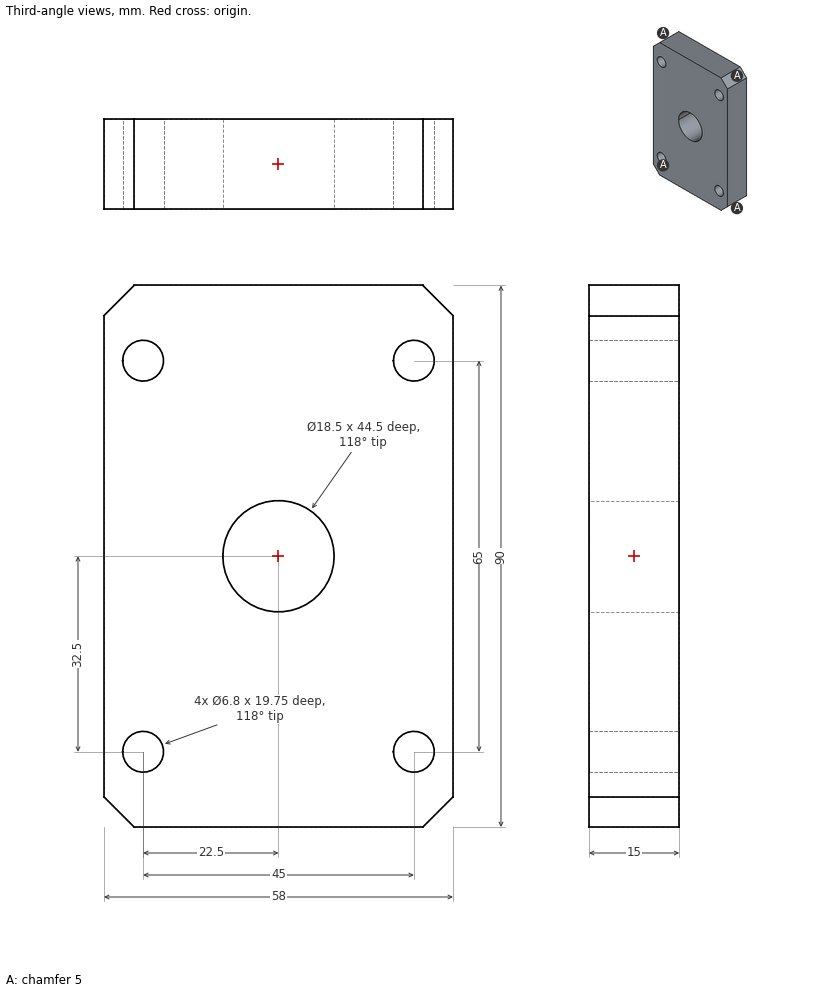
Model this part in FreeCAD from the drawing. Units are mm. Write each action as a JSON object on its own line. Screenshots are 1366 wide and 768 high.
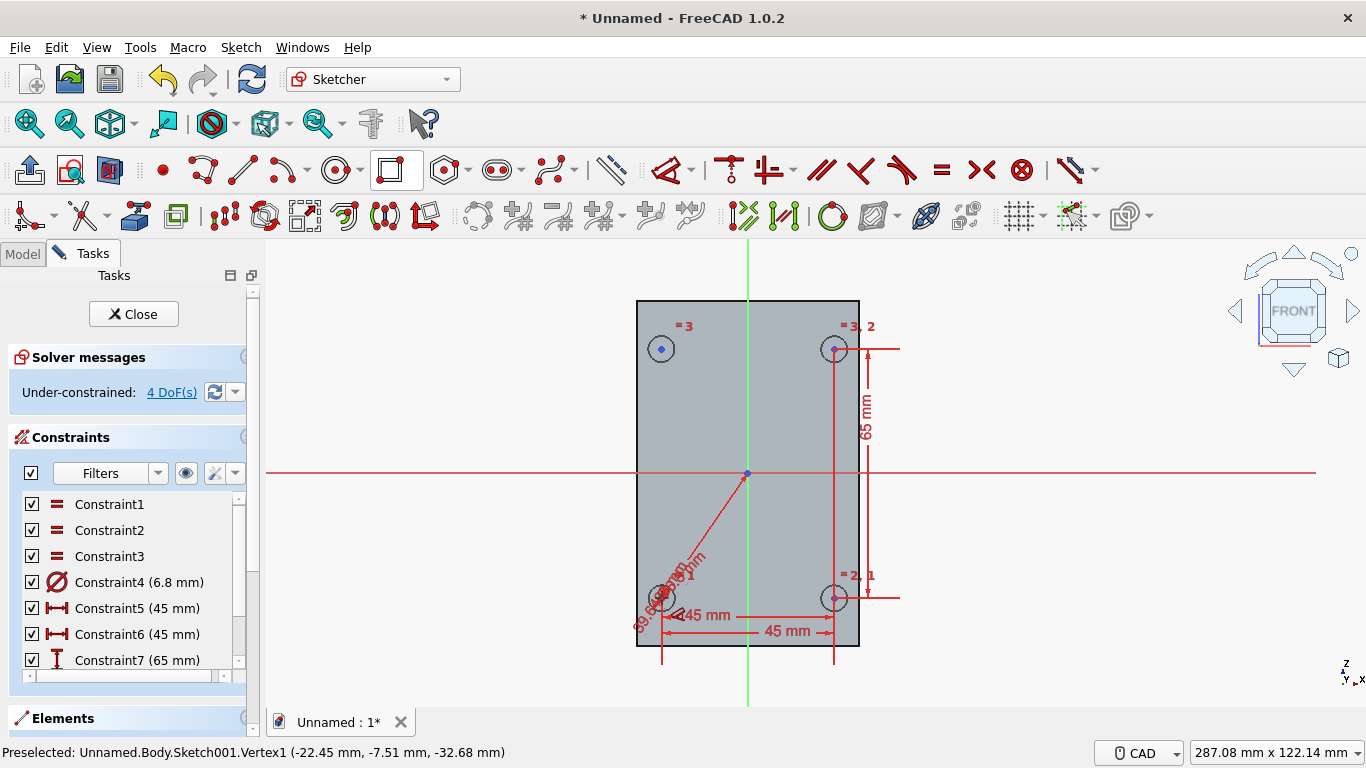
{"action": "left_click", "coordinate": [834, 349]}
{"action": "left_click", "coordinate": [868, 531]}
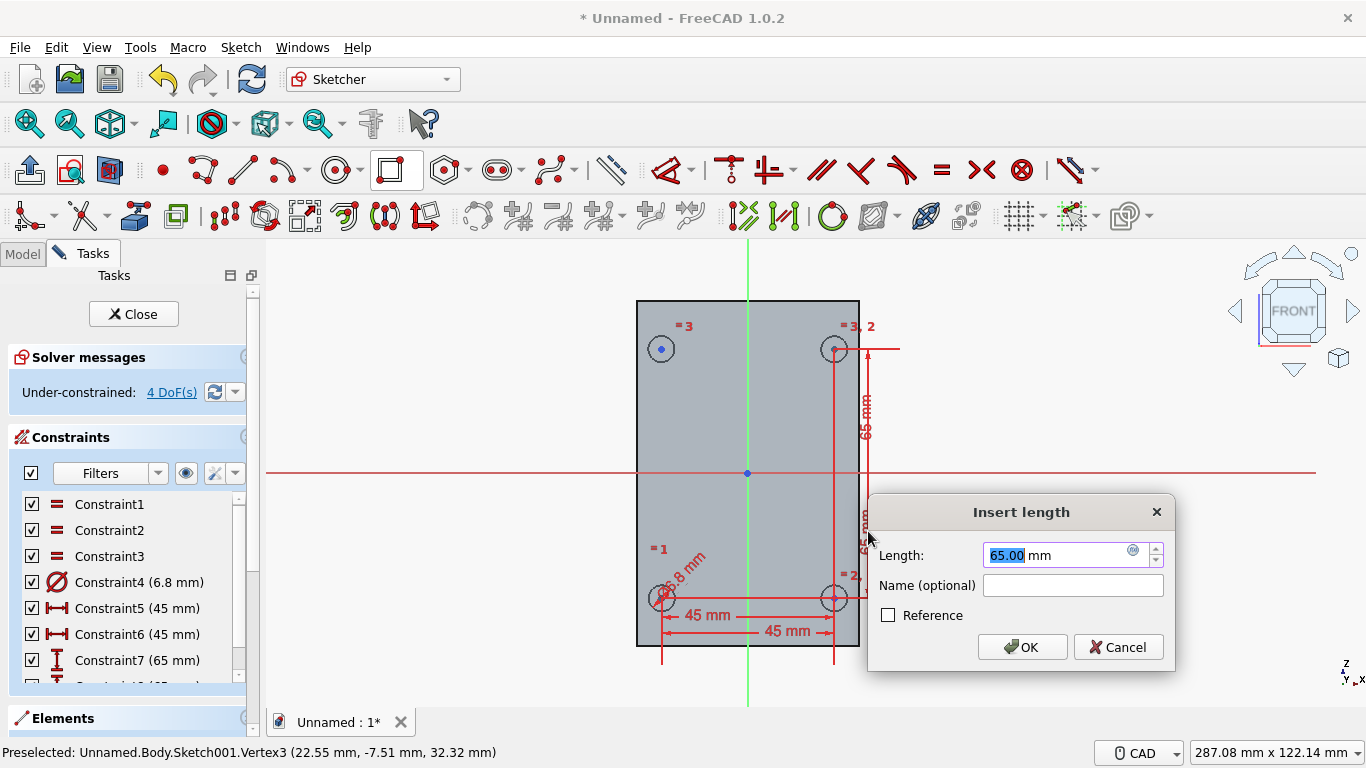
{"action": "type", "text": "65"}
{"action": "key", "text": "Return"}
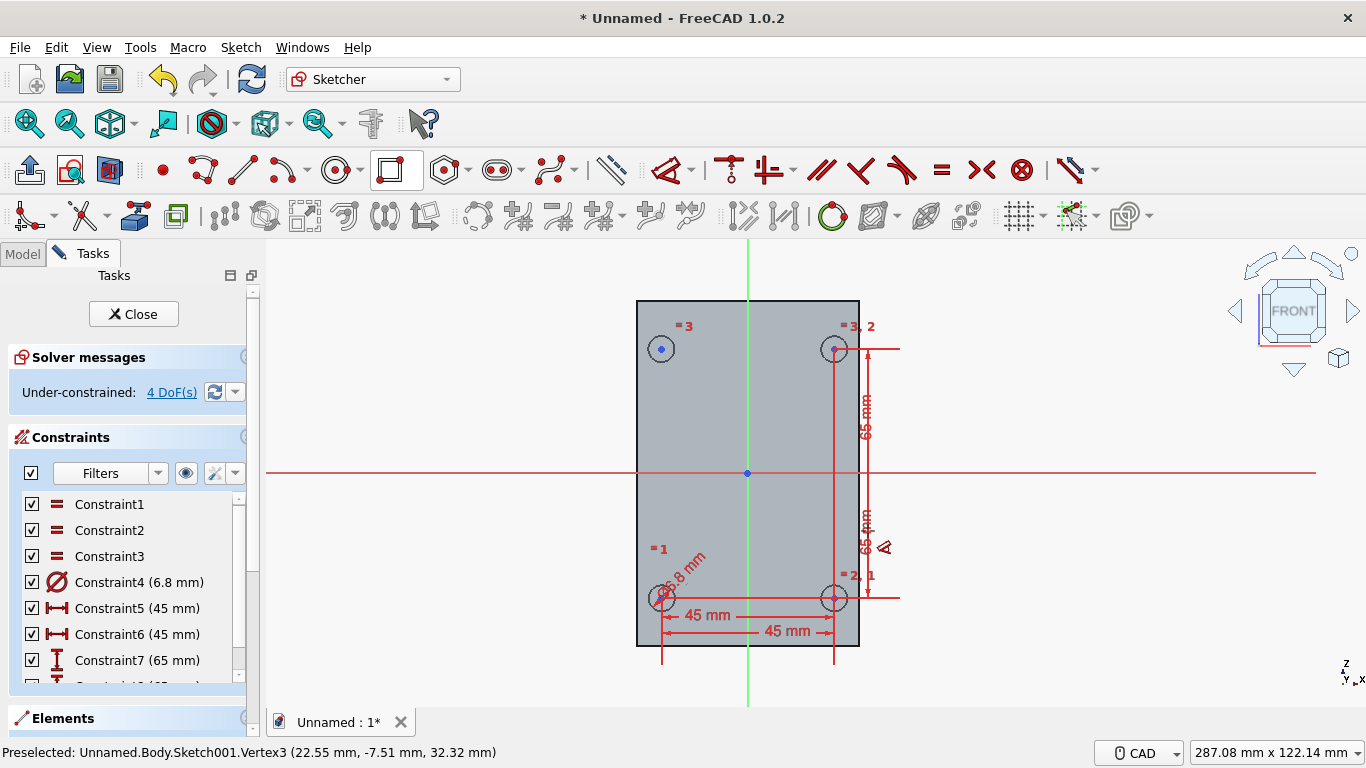
{"action": "left_click", "coordinate": [834, 349]}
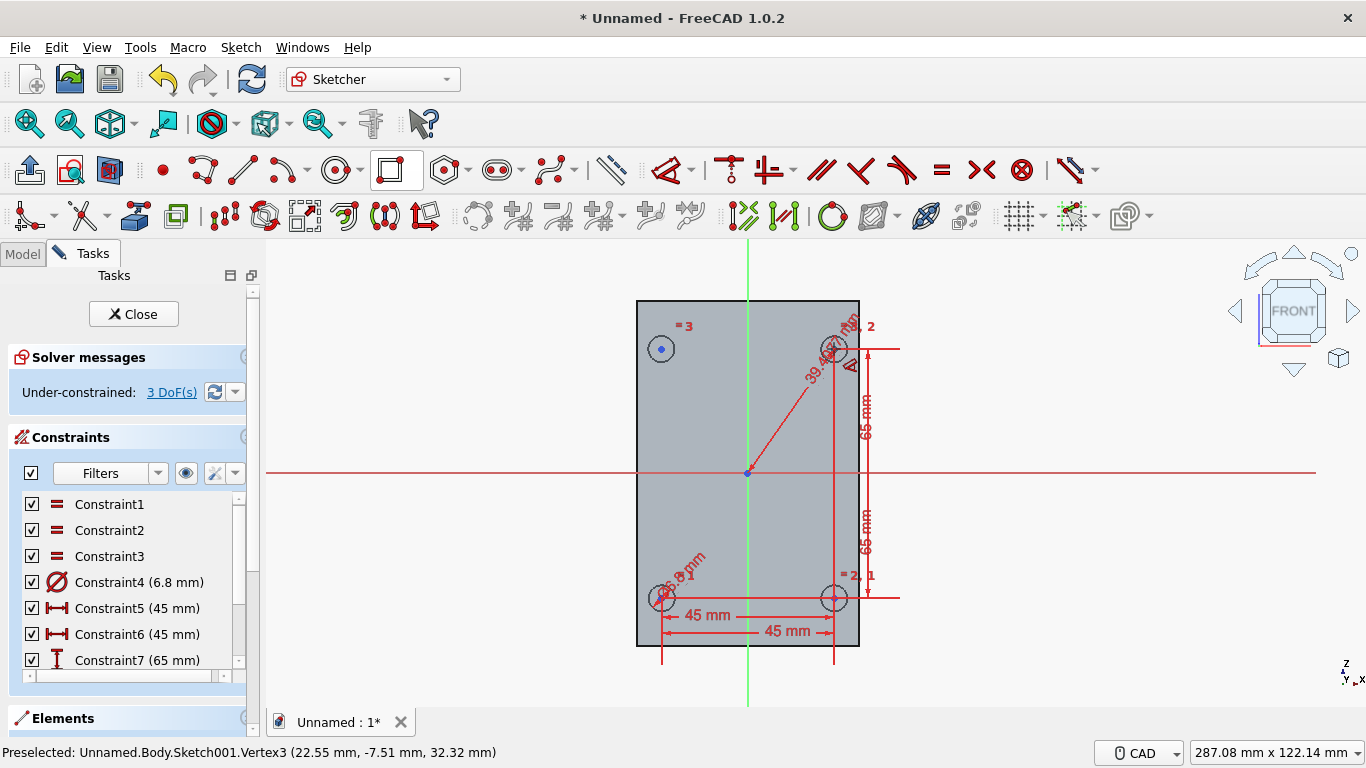
{"action": "left_click", "coordinate": [661, 349]}
{"action": "left_click", "coordinate": [708, 315]}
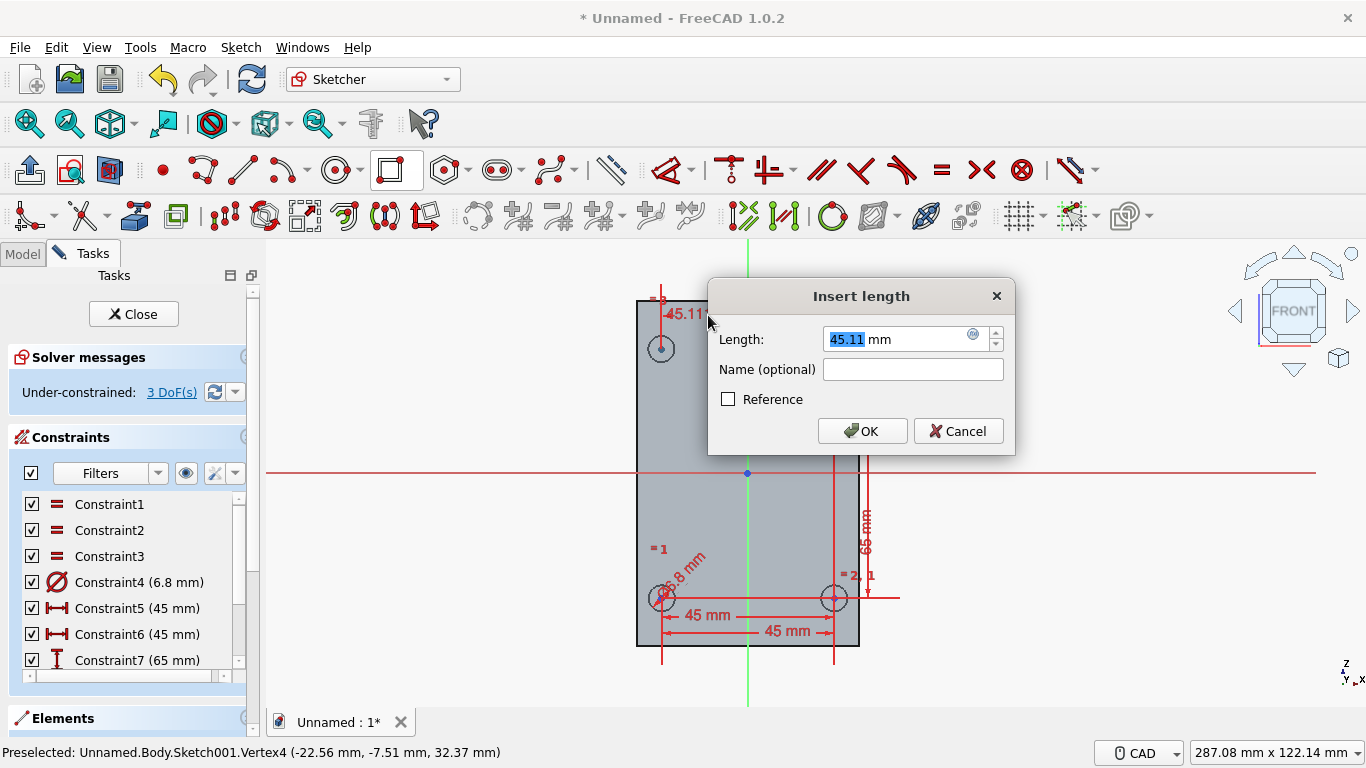
{"action": "type", "text": "45"}
{"action": "key", "text": "Return"}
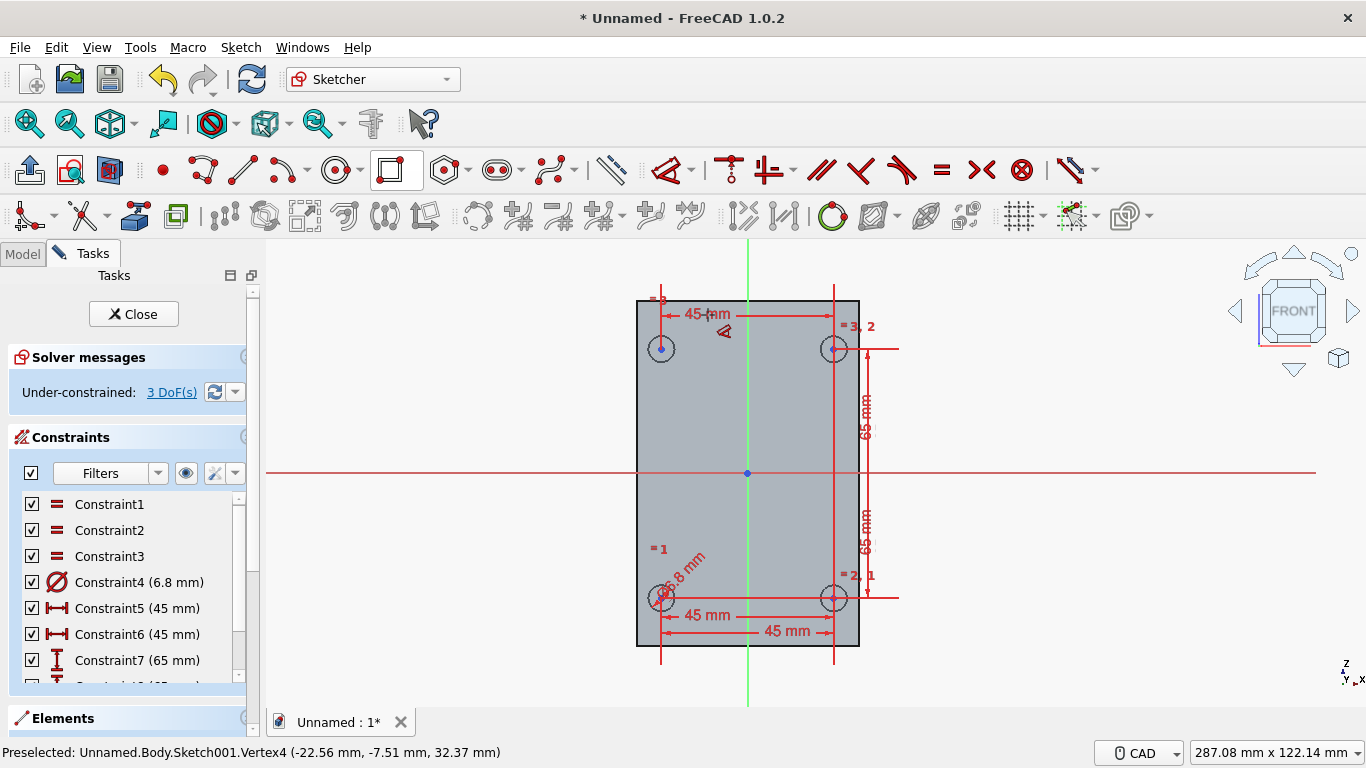
{"action": "left_click", "coordinate": [661, 598]}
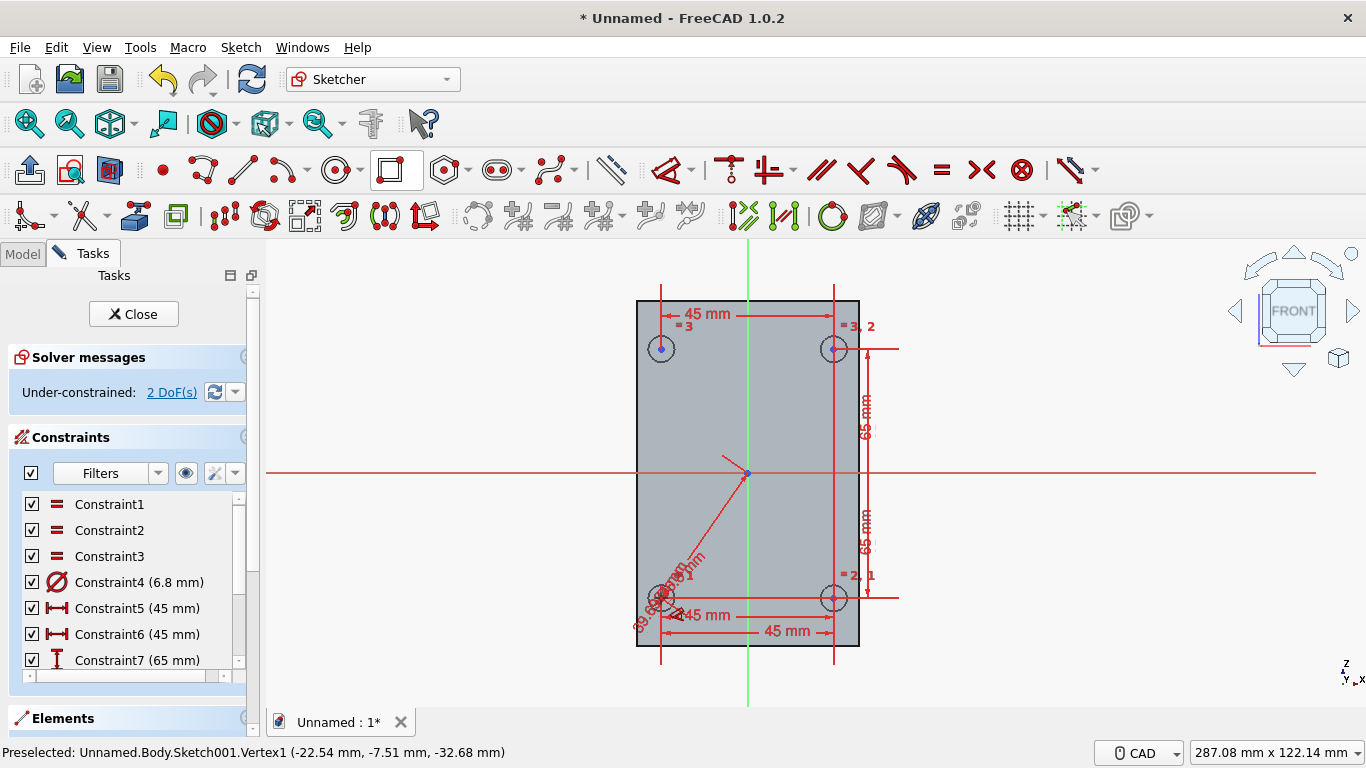
{"action": "left_click", "coordinate": [661, 349]}
{"action": "left_click", "coordinate": [627, 416]}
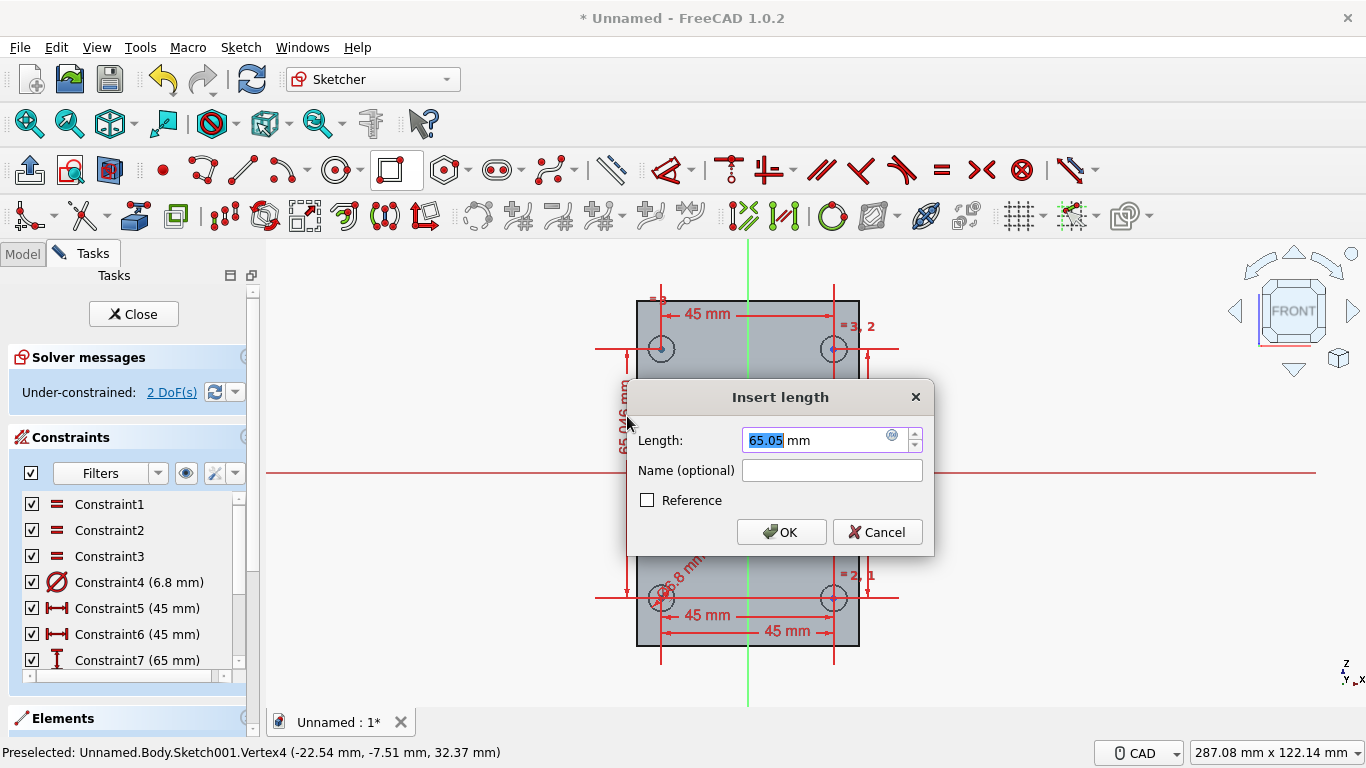
{"action": "type", "text": "65"}
{"action": "key", "text": "Return"}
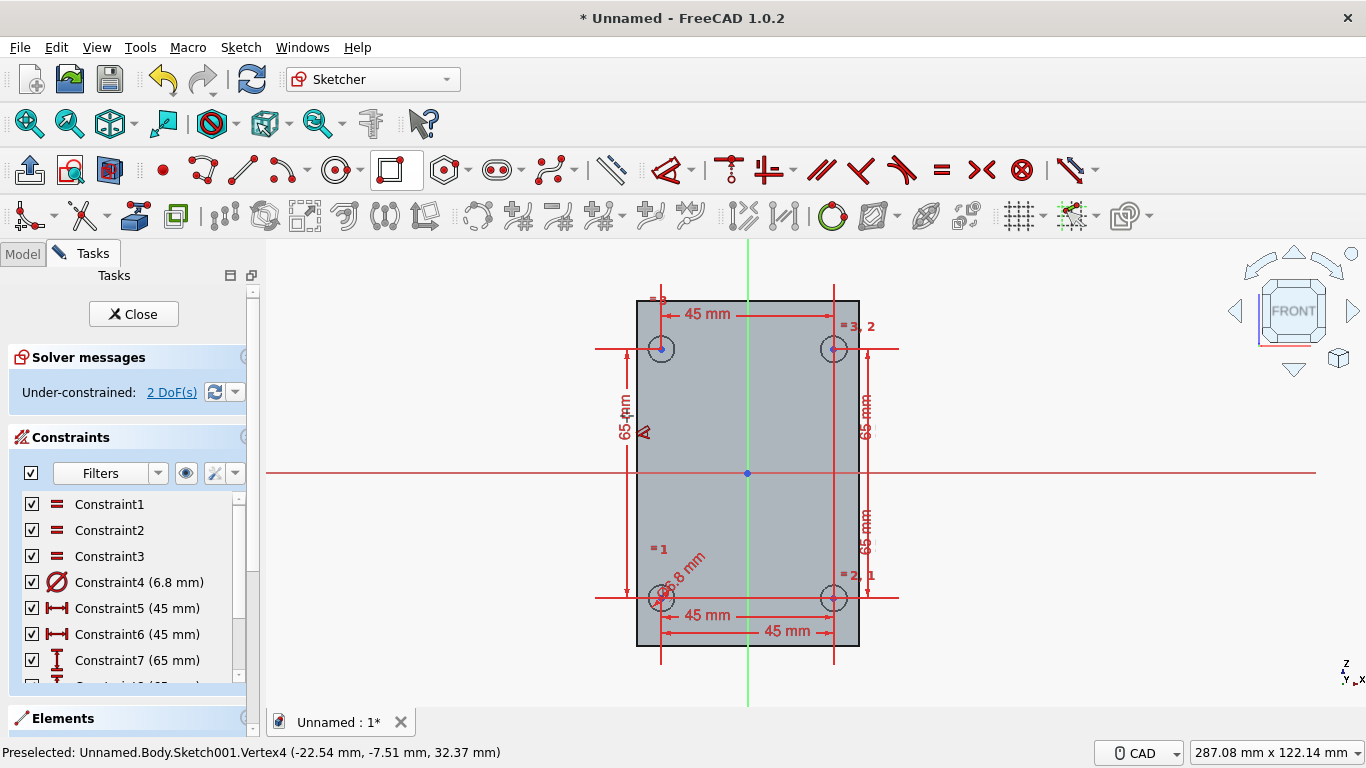
{"action": "left_click", "coordinate": [661, 598]}
{"action": "left_click", "coordinate": [705, 439]}